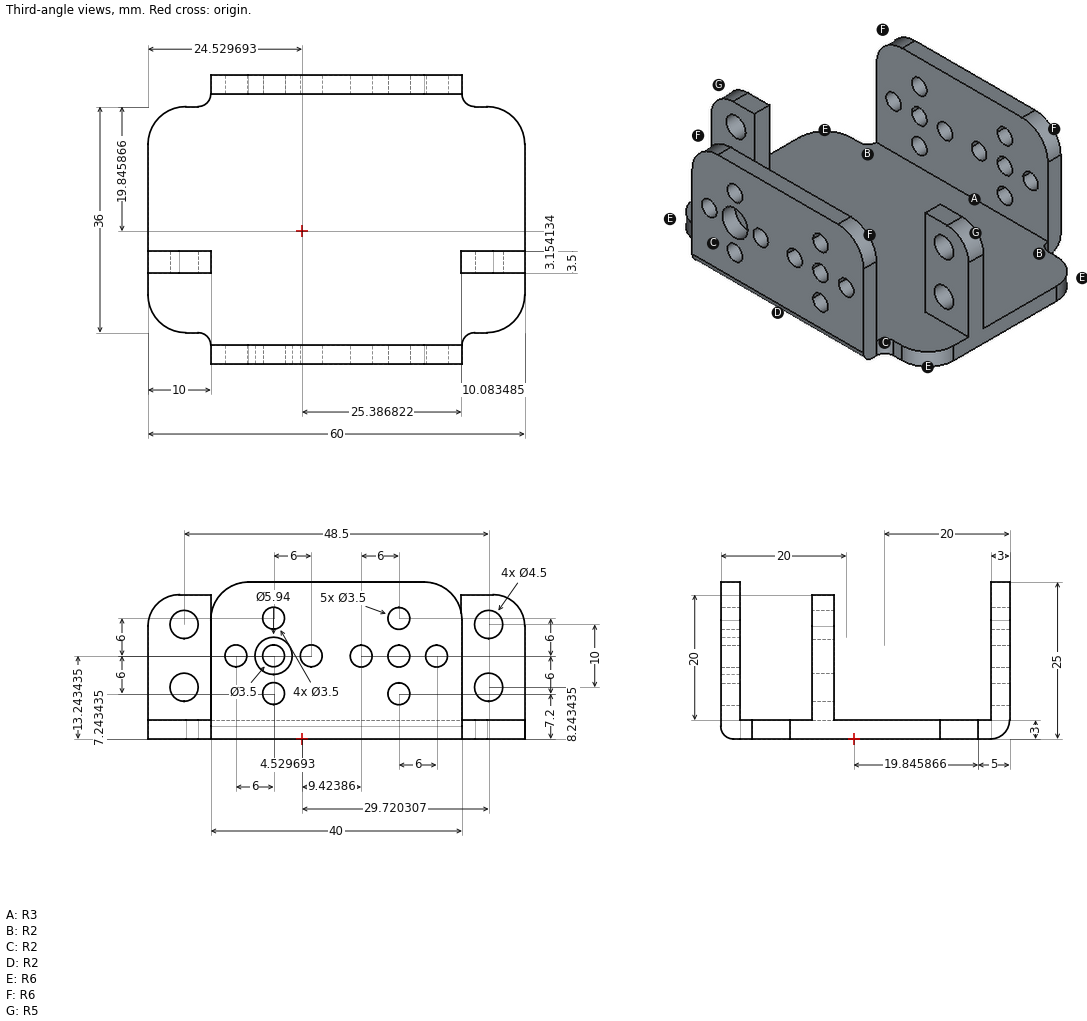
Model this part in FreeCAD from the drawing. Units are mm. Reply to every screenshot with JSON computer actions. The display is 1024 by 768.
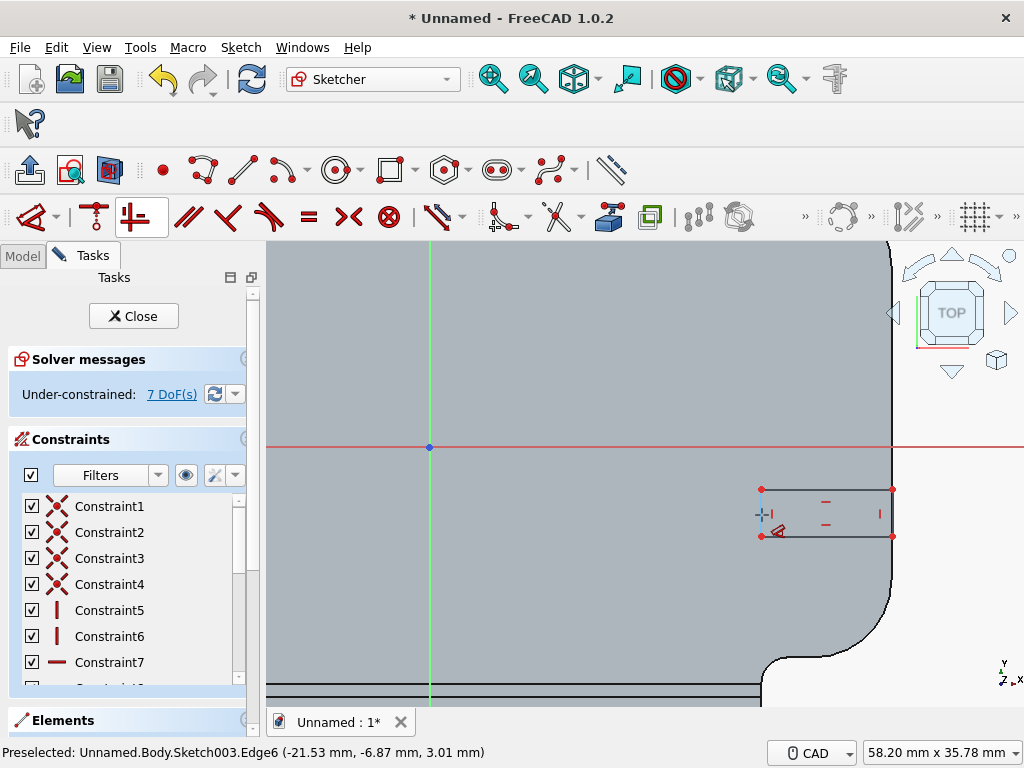
{"action": "left_click", "coordinate": [761, 513]}
{"action": "left_click", "coordinate": [795, 513]}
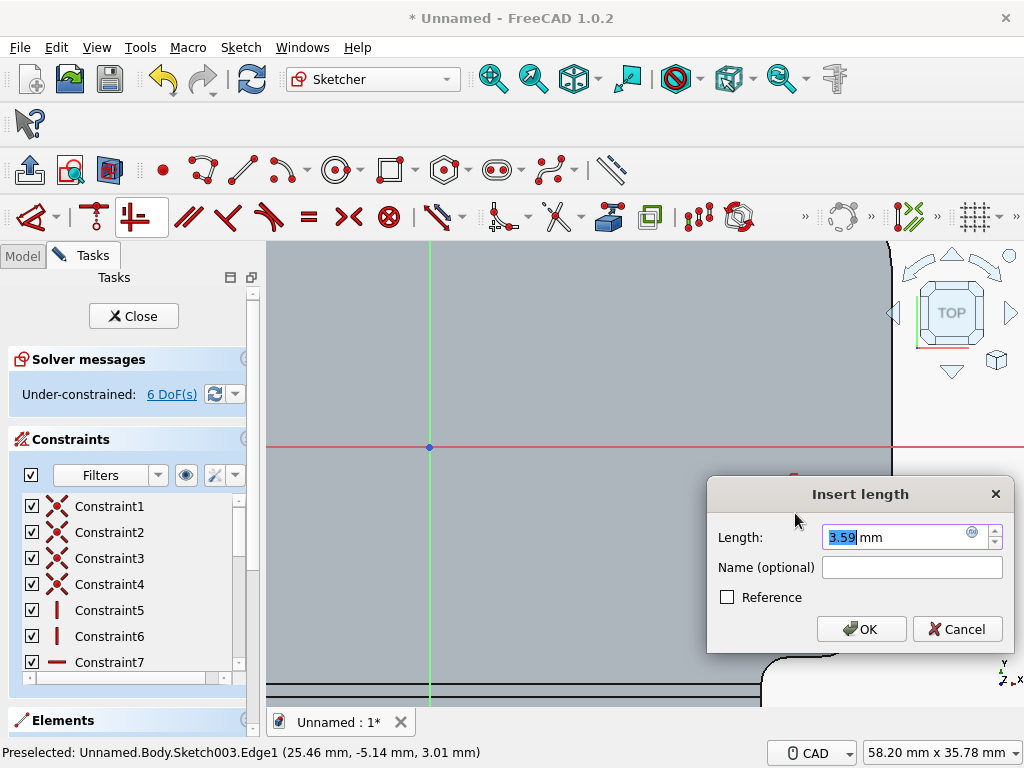
{"action": "type", "text": "3.5"}
{"action": "key", "text": "Return"}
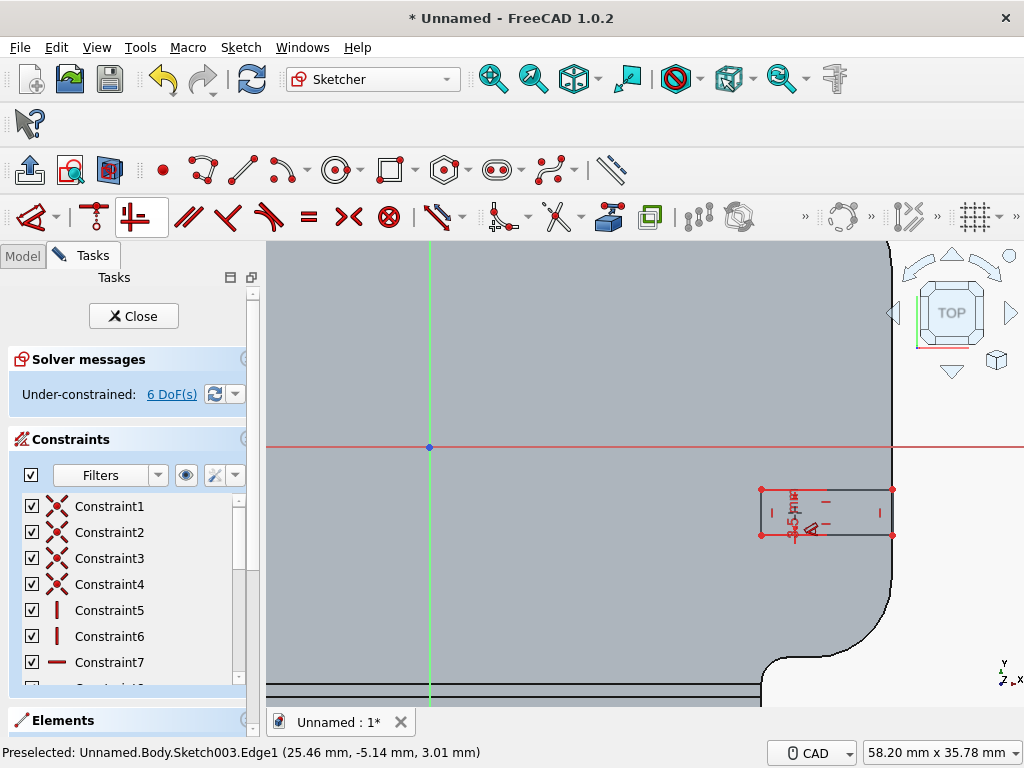
{"action": "scroll", "coordinate": [669, 454], "scroll_direction": "down", "scroll_amount": 3}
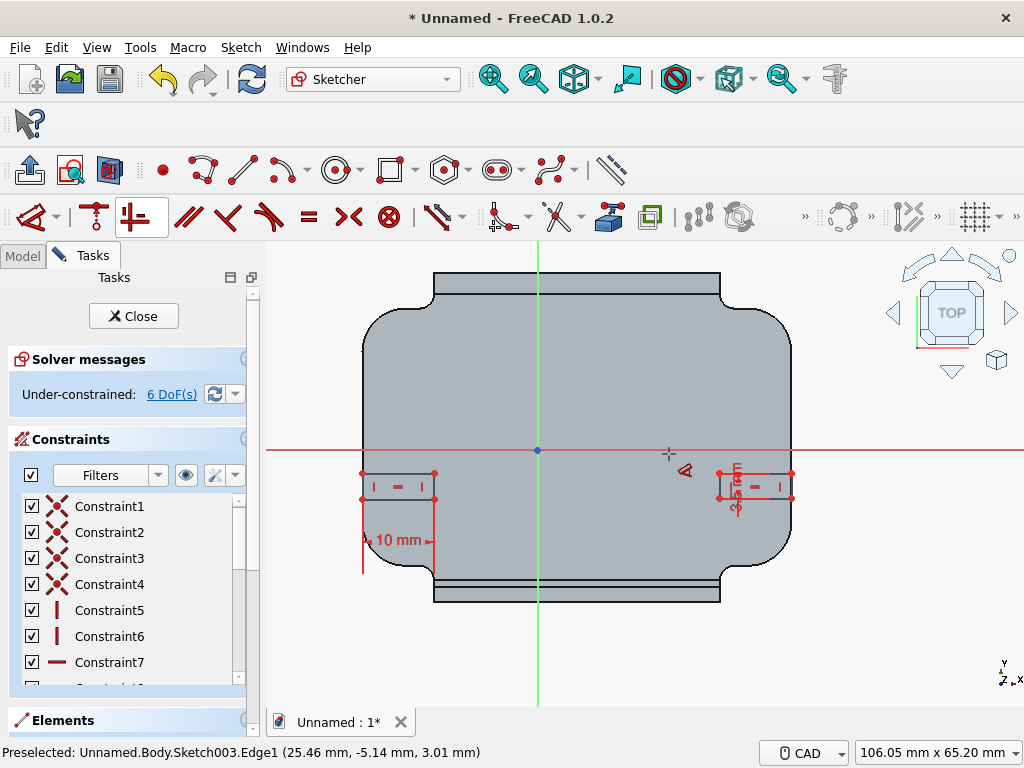
{"action": "scroll", "coordinate": [363, 482], "scroll_direction": "up", "scroll_amount": 3}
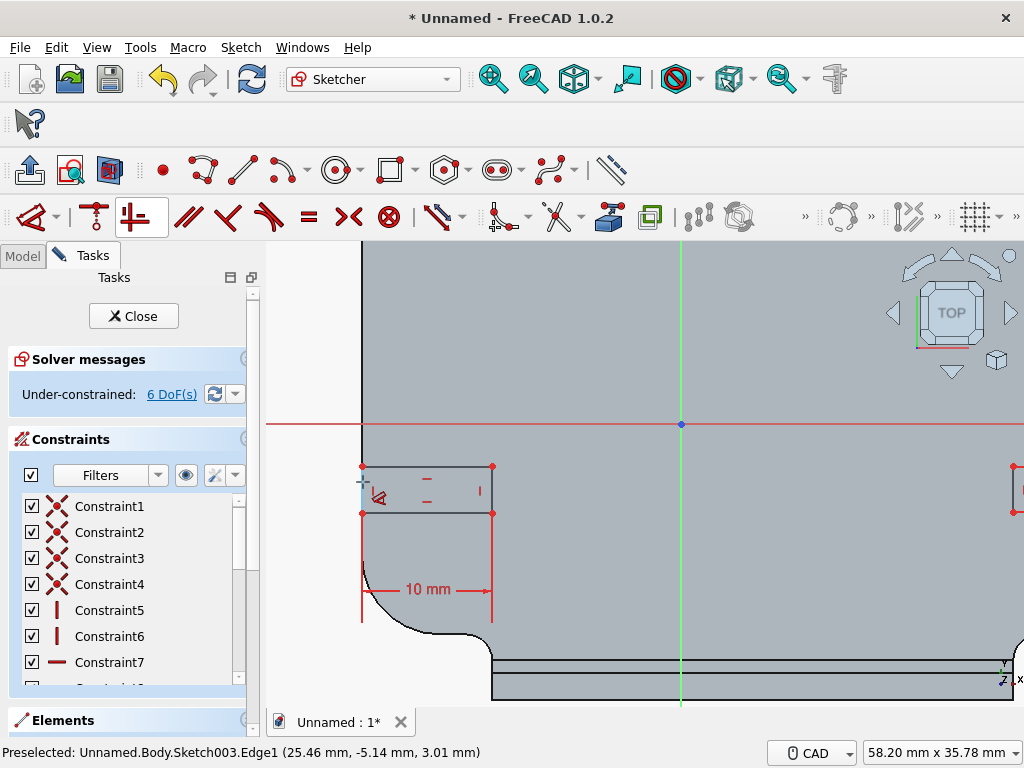
{"action": "left_click", "coordinate": [362, 481]}
{"action": "left_click", "coordinate": [328, 490]}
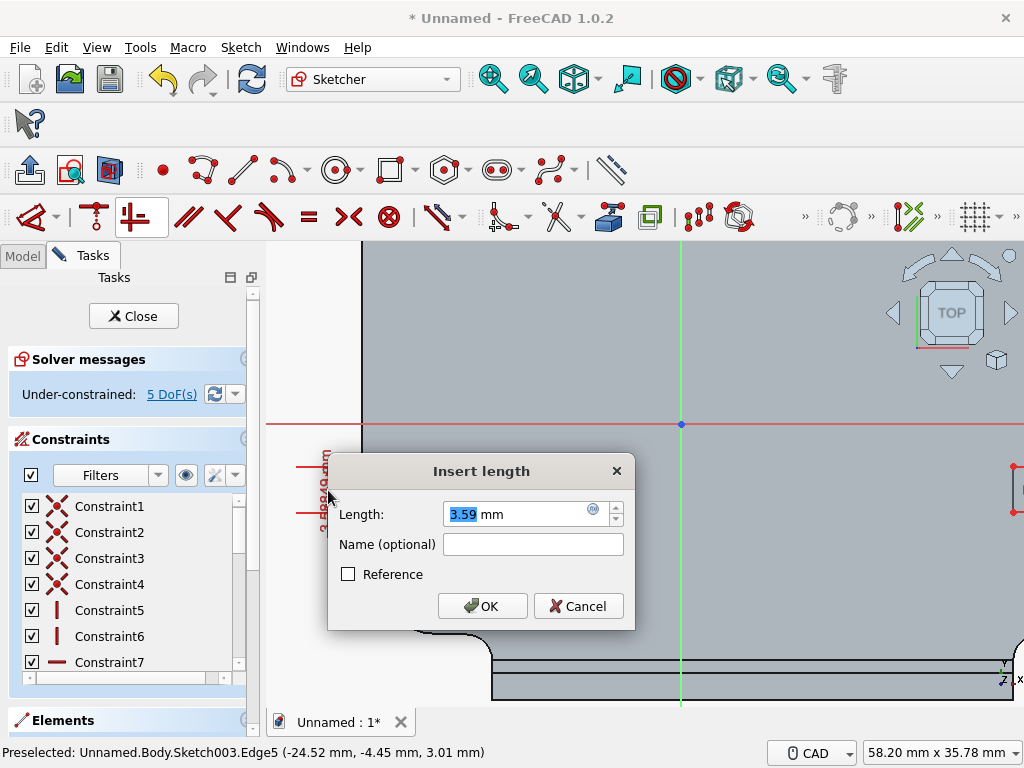
{"action": "type", "text": "3.5"}
{"action": "key", "text": "Return"}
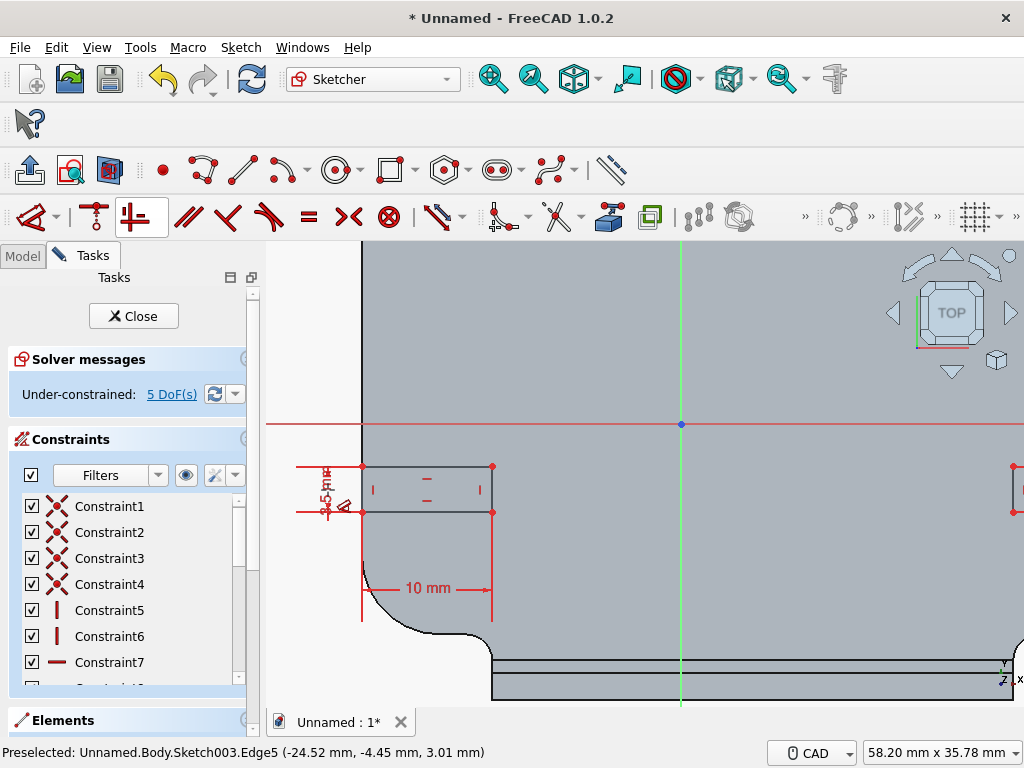
{"action": "scroll", "coordinate": [362, 482], "scroll_direction": "down", "scroll_amount": 3}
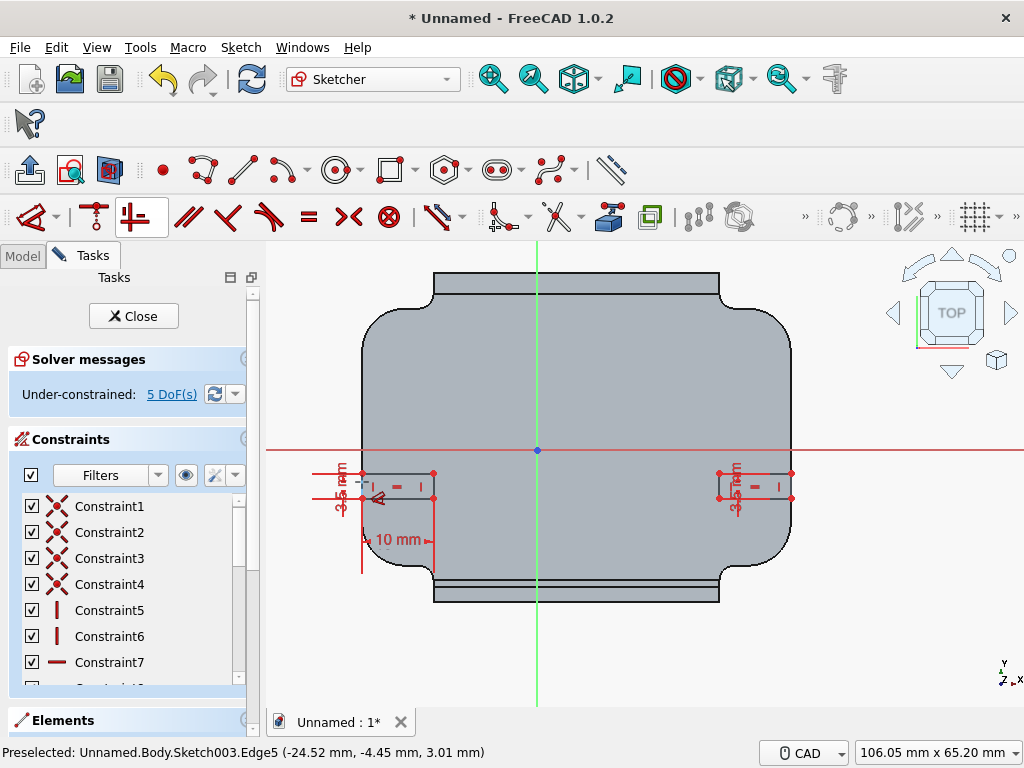
{"action": "left_click", "coordinate": [741, 499]}
{"action": "left_click", "coordinate": [755, 533]}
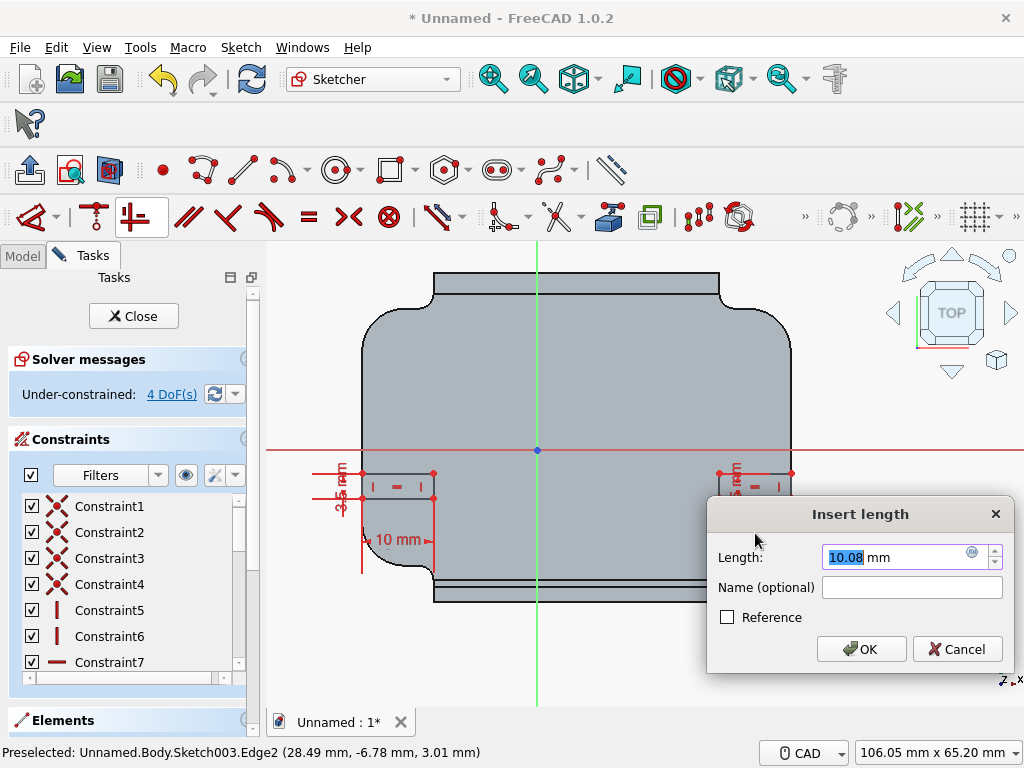
{"action": "type", "text": "10.083485"}
{"action": "key", "text": "Return"}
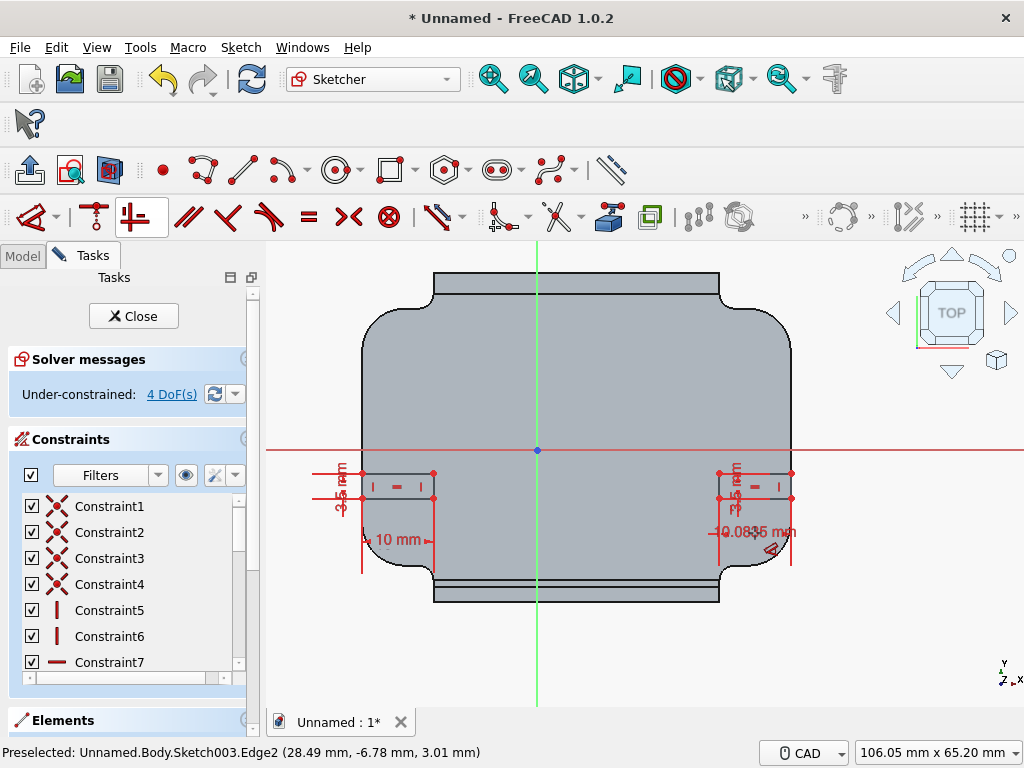
{"action": "scroll", "coordinate": [719, 474], "scroll_direction": "up", "scroll_amount": 3}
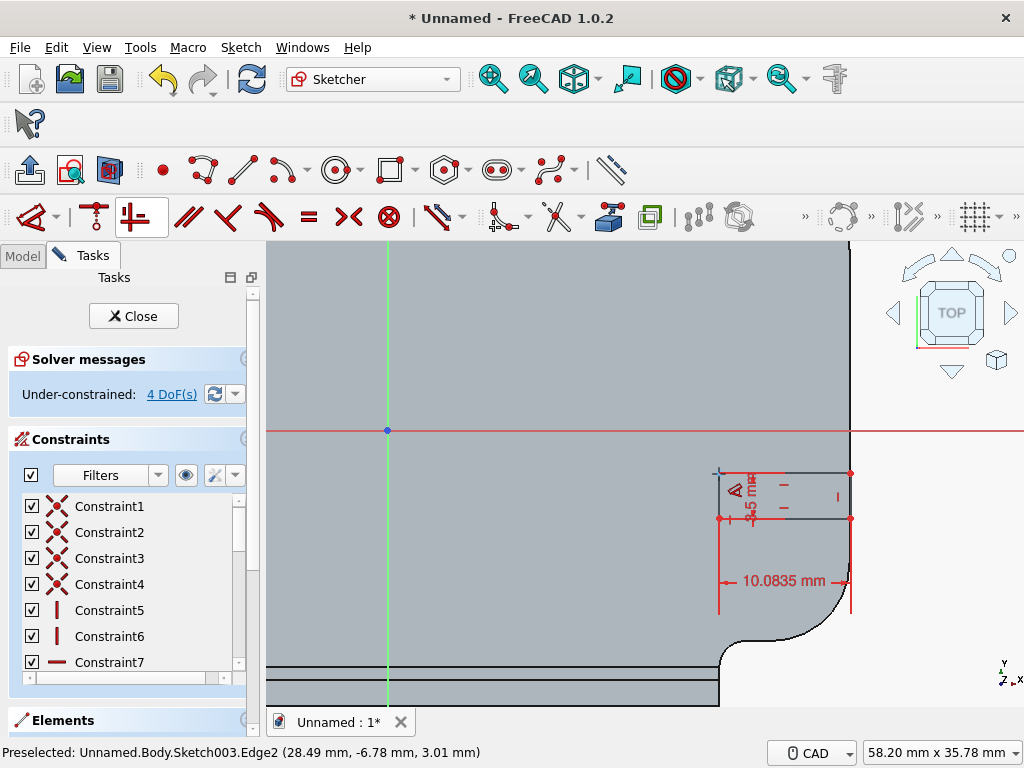
{"action": "left_click", "coordinate": [719, 473]}
{"action": "left_click", "coordinate": [753, 452]}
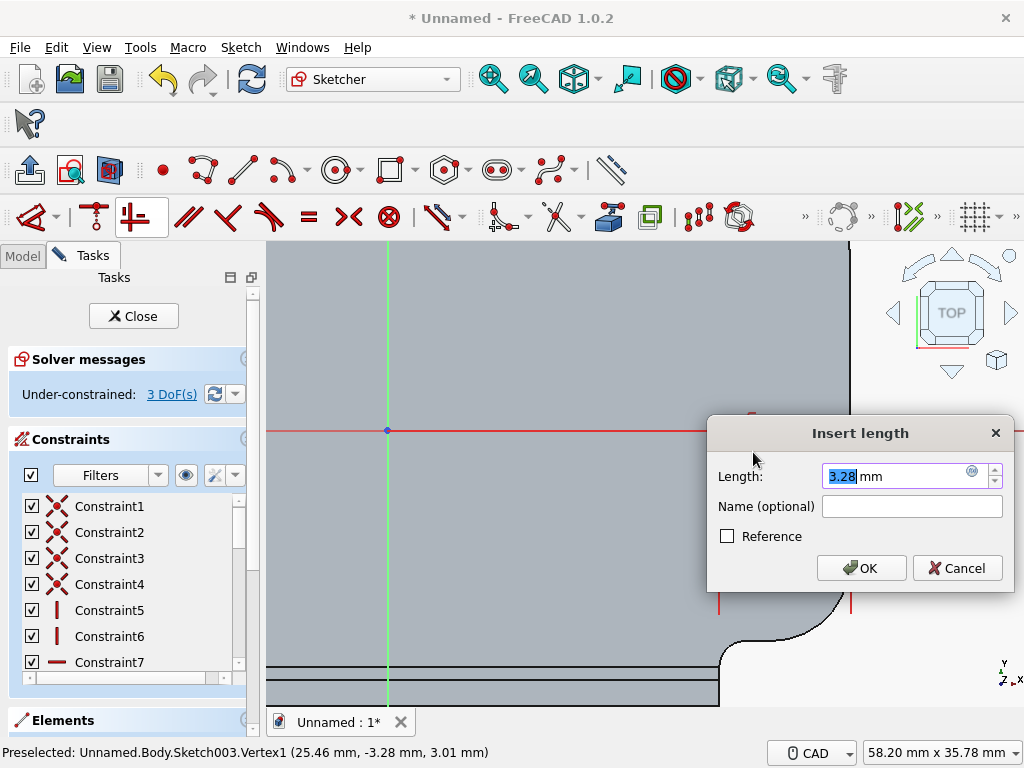
{"action": "type", "text": "3.154134"}
{"action": "key", "text": "Return"}